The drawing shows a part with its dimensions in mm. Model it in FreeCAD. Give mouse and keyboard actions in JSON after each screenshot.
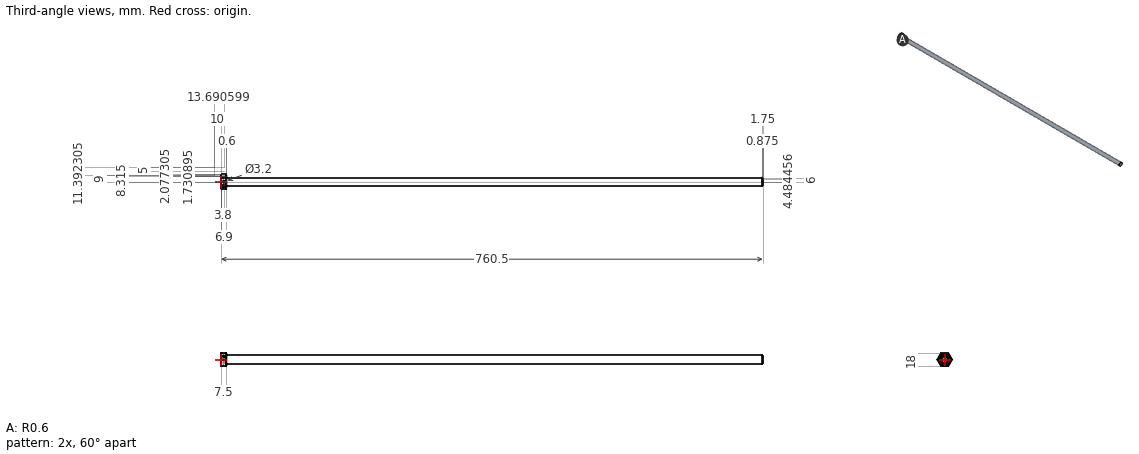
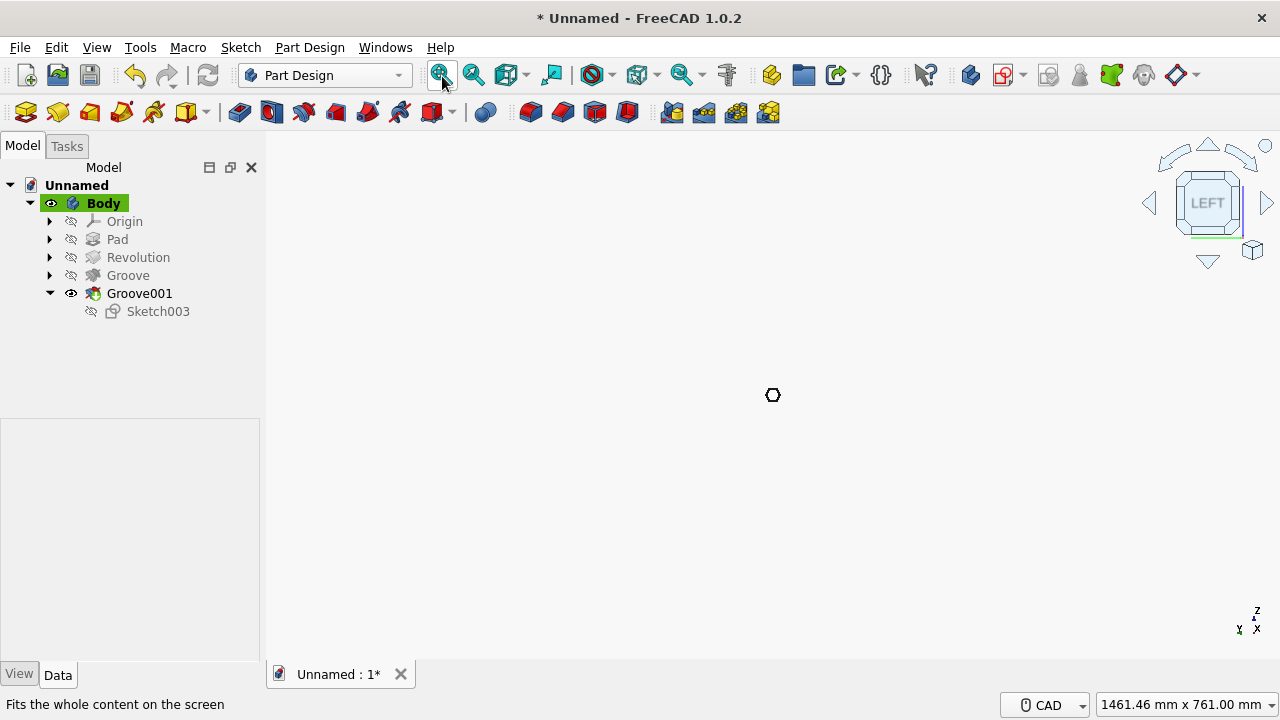
{"action": "key", "text": "v 3"}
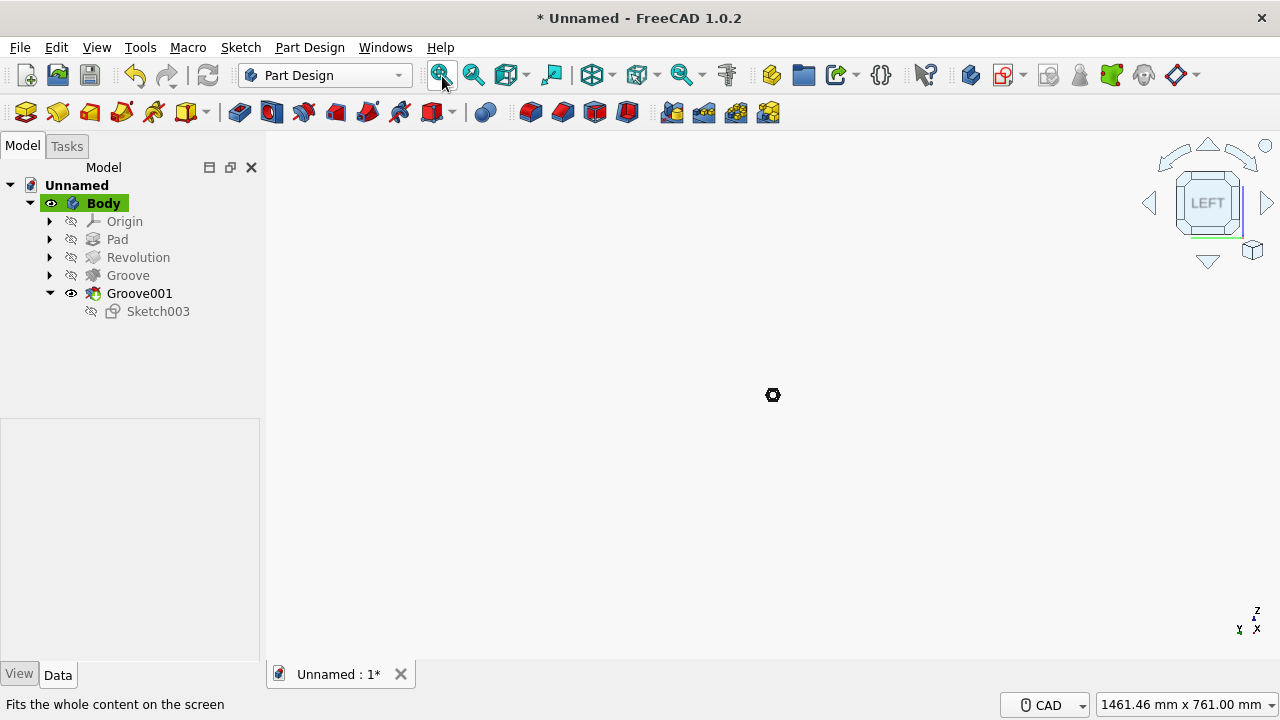
{"action": "key", "text": "0"}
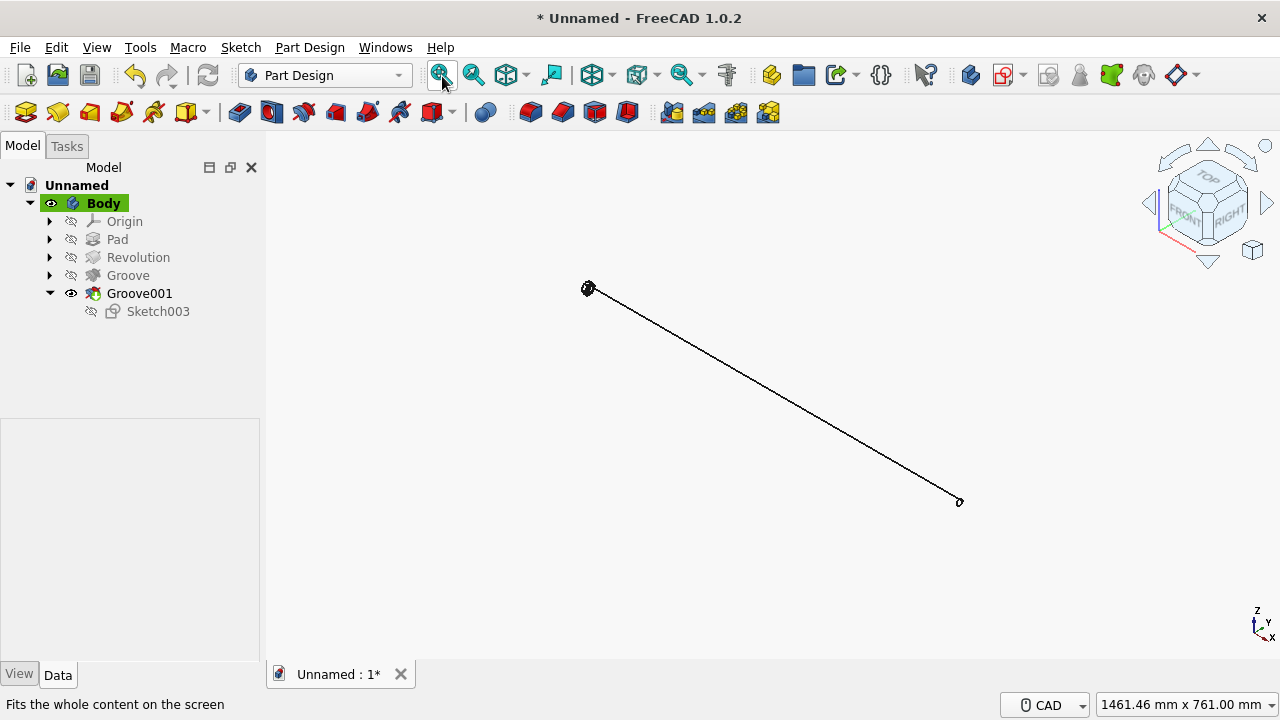
{"action": "left_click", "coordinate": [442, 76]}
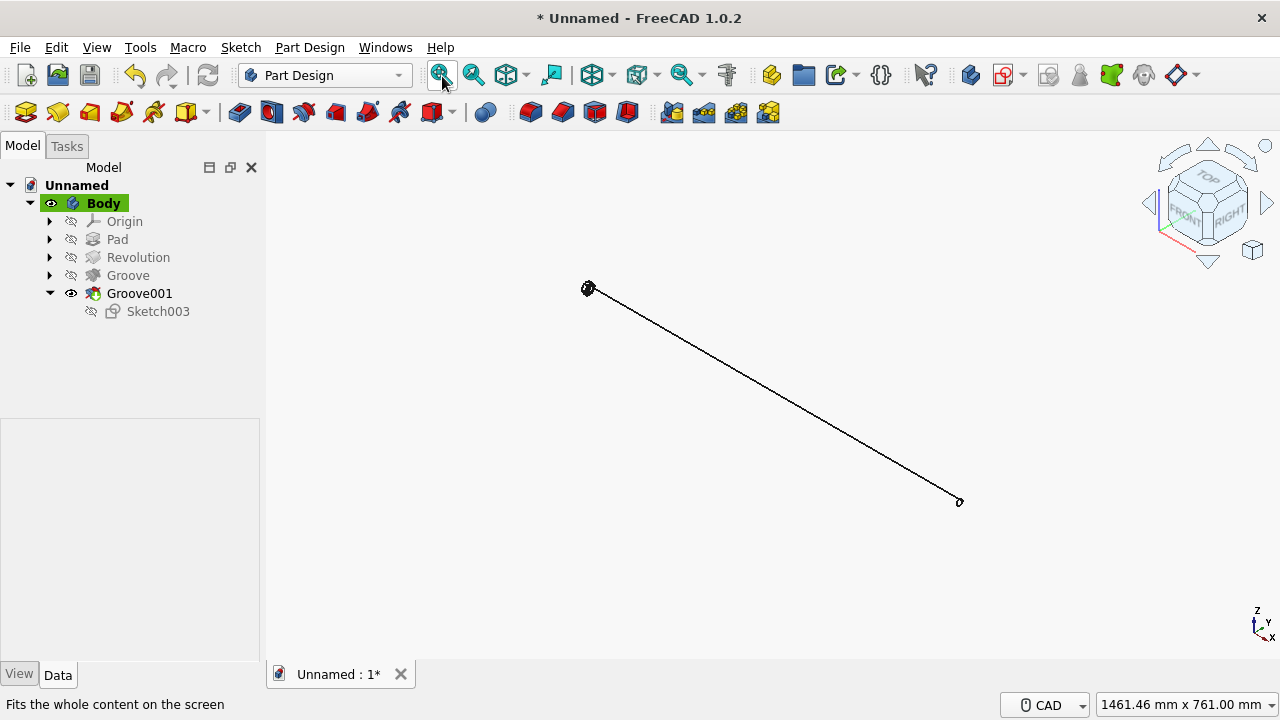
{"action": "scroll", "coordinate": [587, 290], "scroll_direction": "up", "scroll_amount": 6}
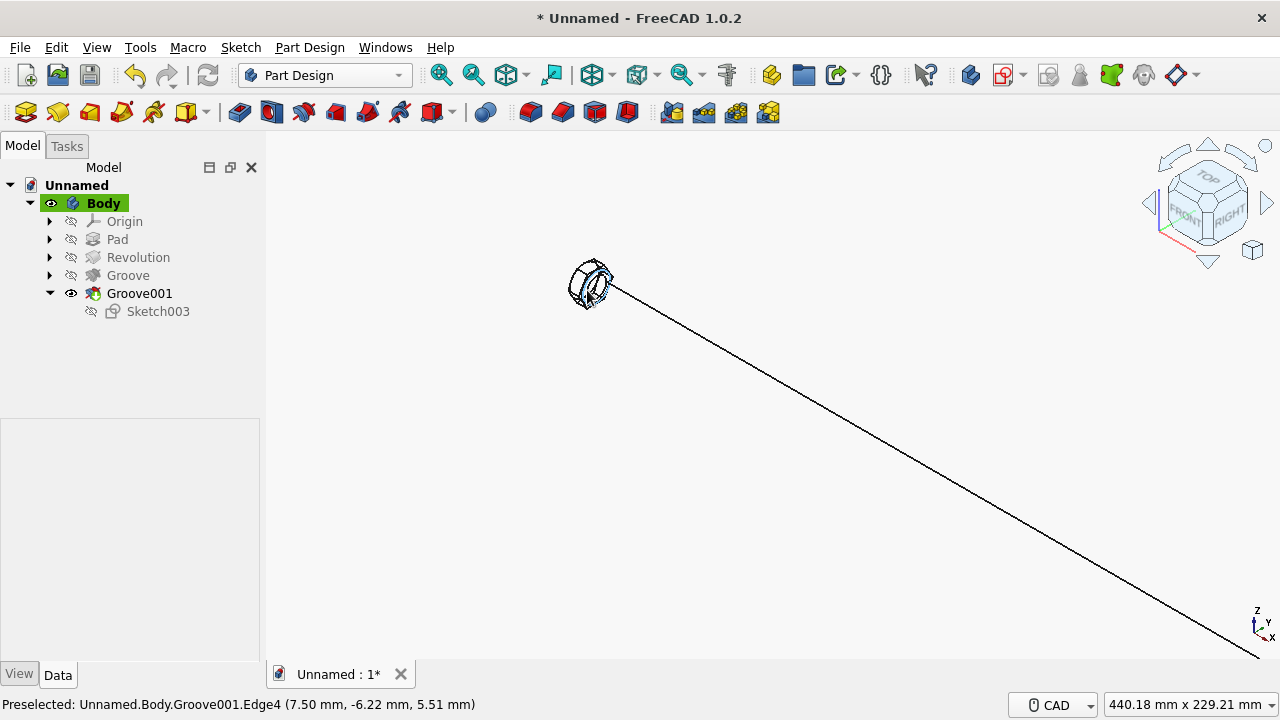
{"action": "left_click", "coordinate": [594, 299]}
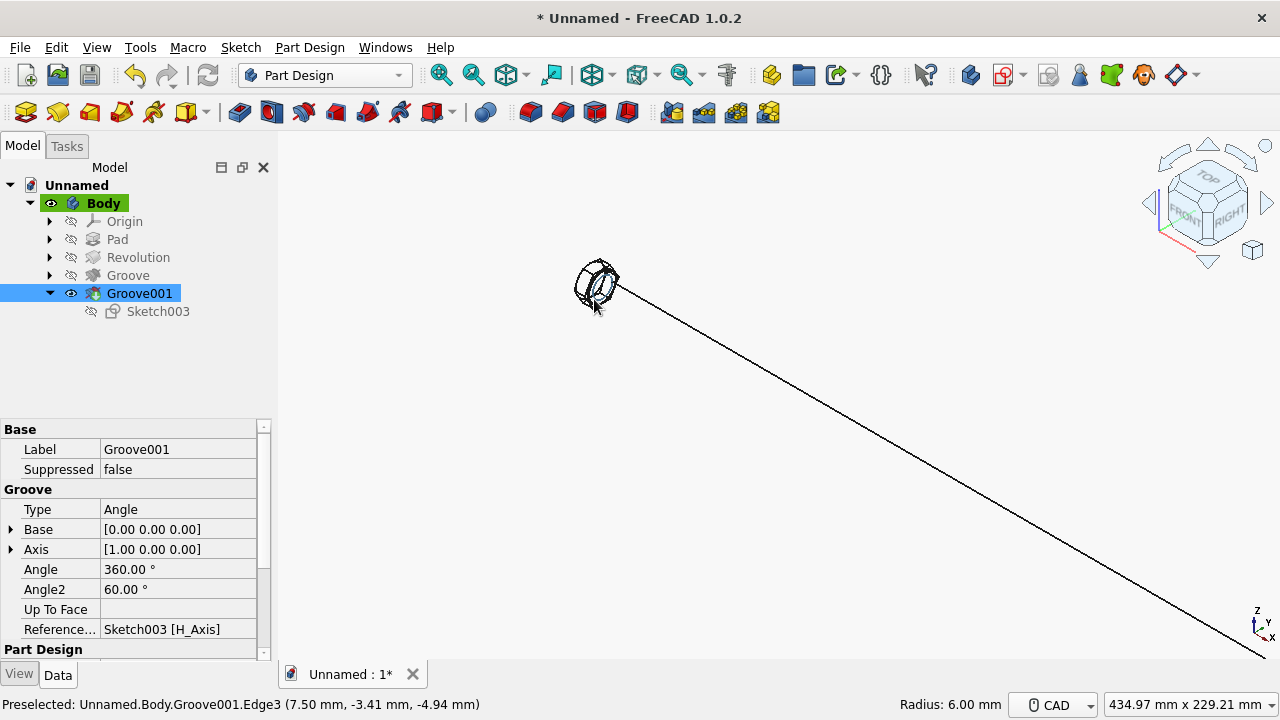
{"action": "key", "text": "v 1"}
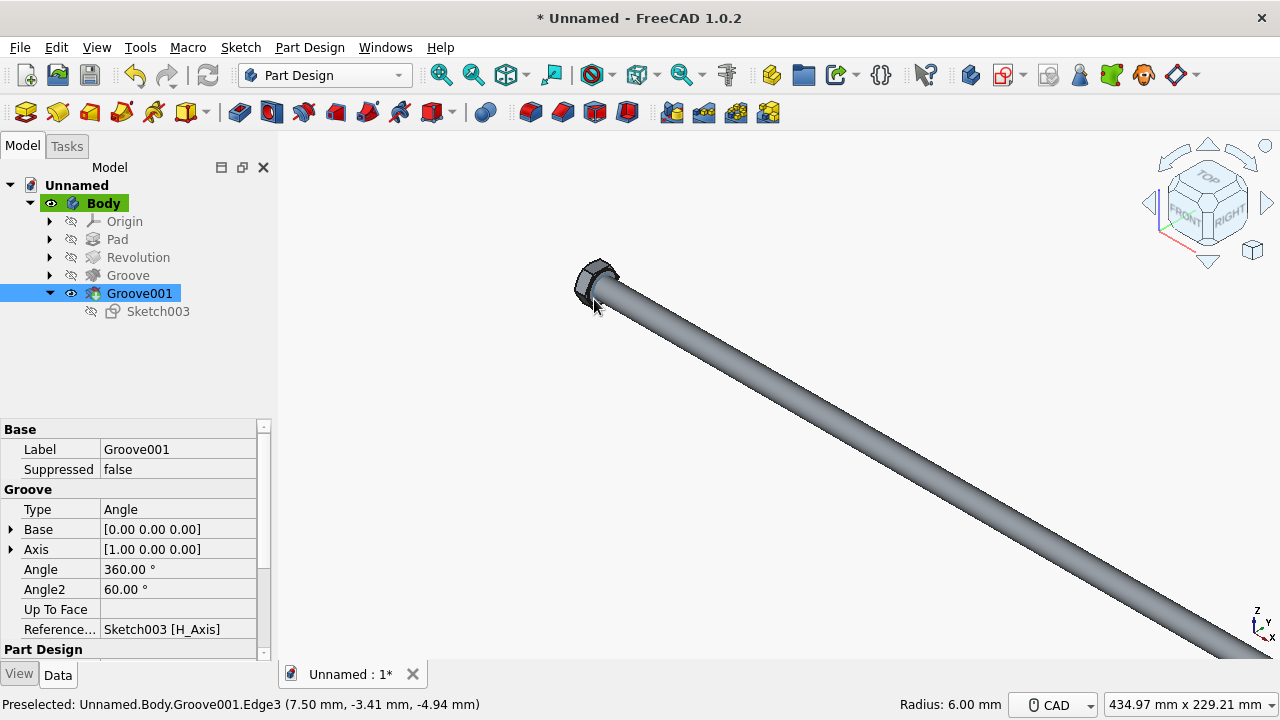
{"action": "left_click", "coordinate": [532, 112]}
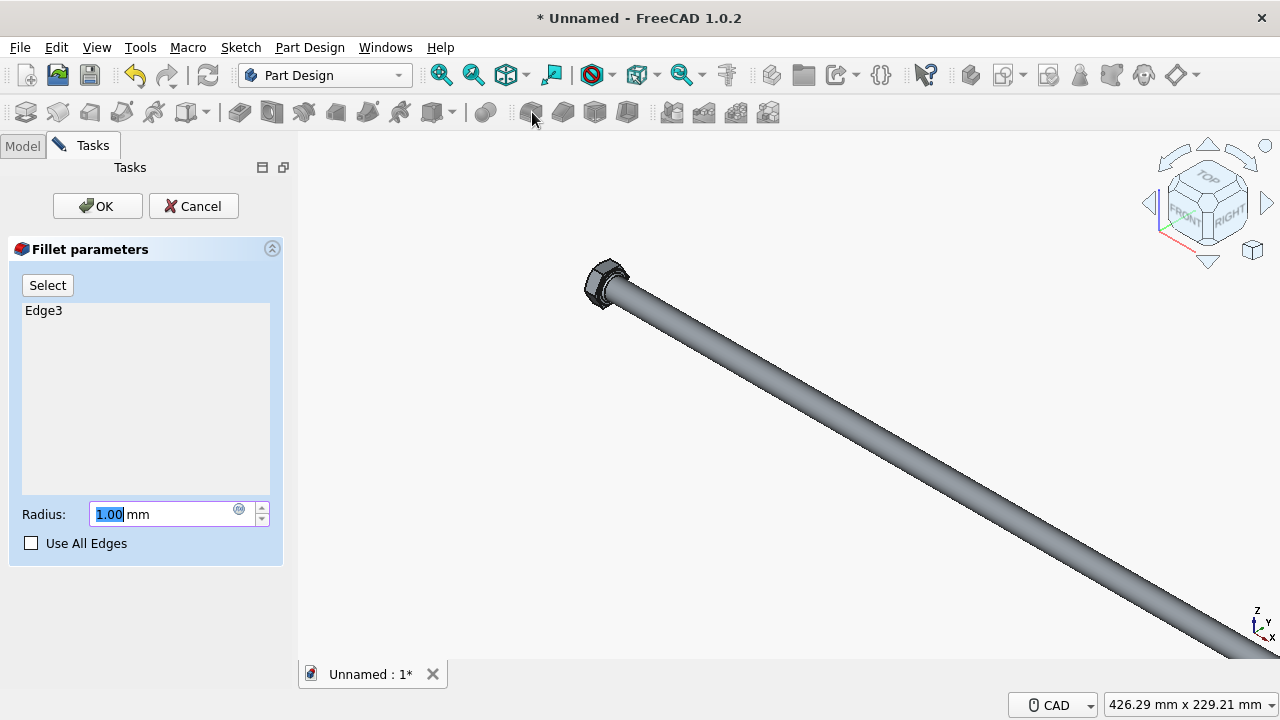
{"action": "type", "text": "0.6"}
{"action": "key", "text": "Tab"}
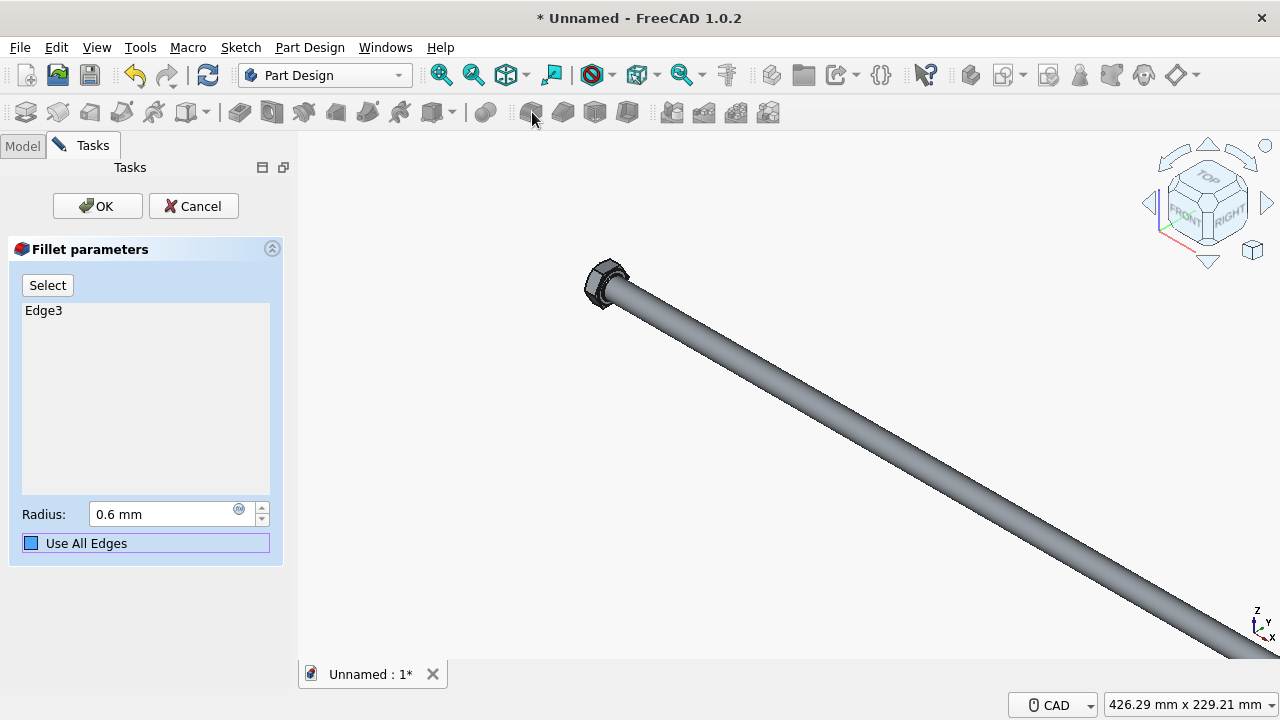
{"action": "left_click", "coordinate": [98, 206]}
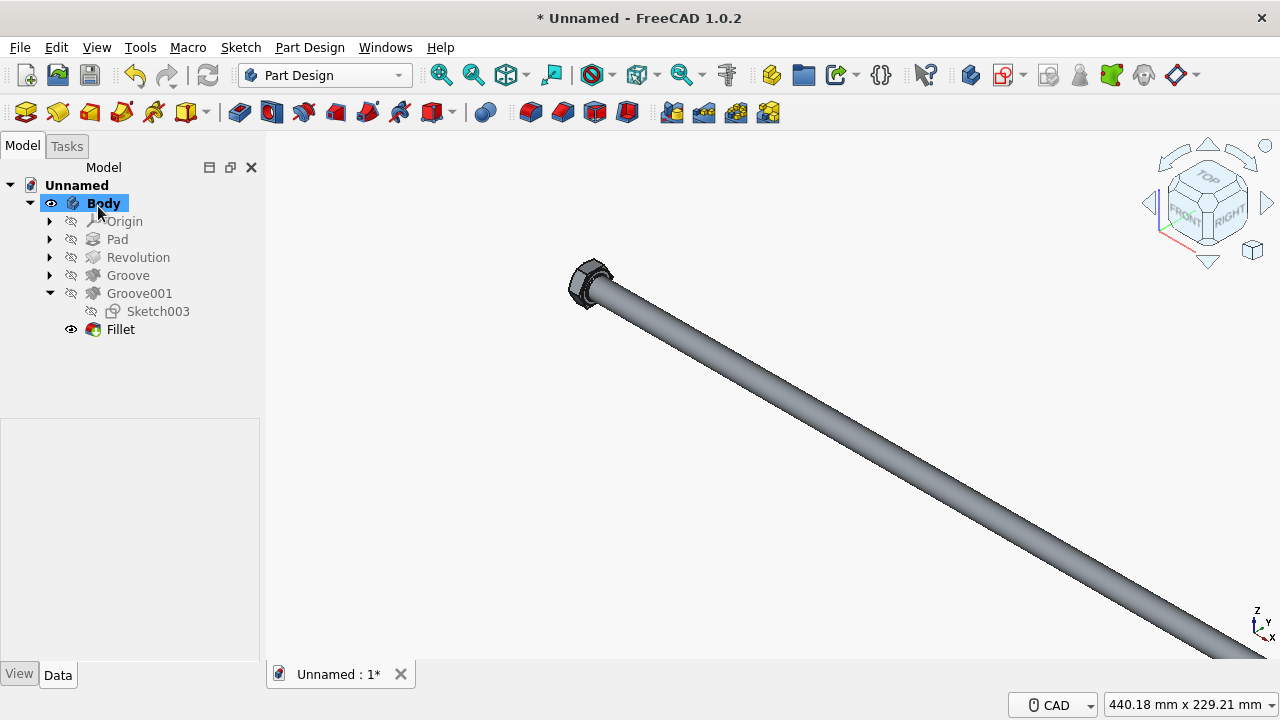
{"action": "key", "text": "v f"}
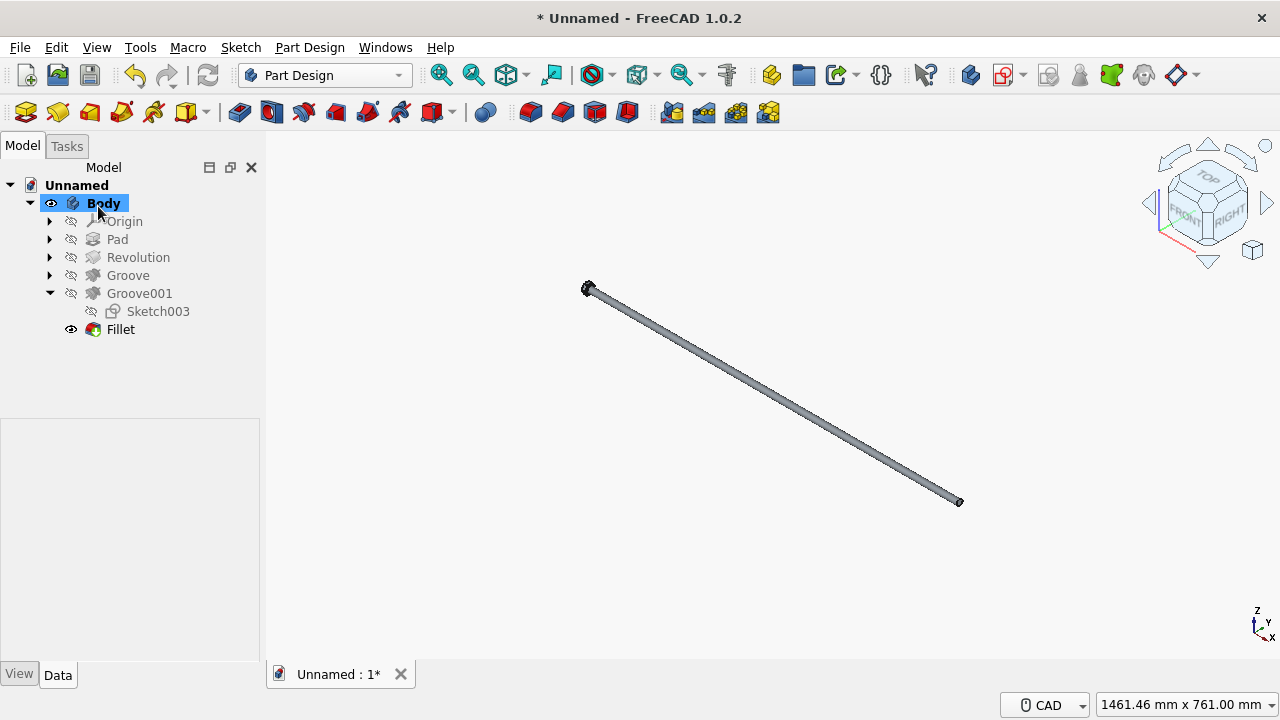
{"action": "left_click", "coordinate": [1004, 76]}